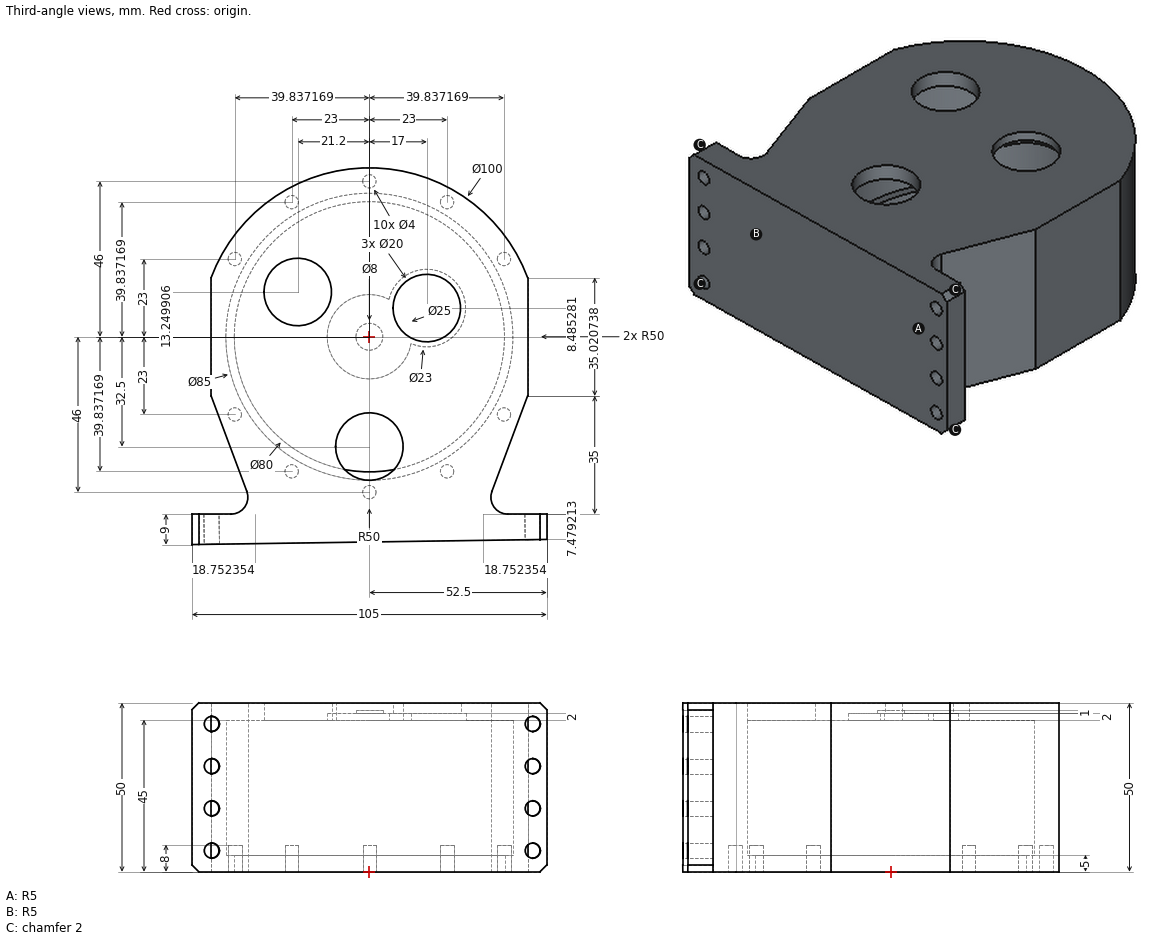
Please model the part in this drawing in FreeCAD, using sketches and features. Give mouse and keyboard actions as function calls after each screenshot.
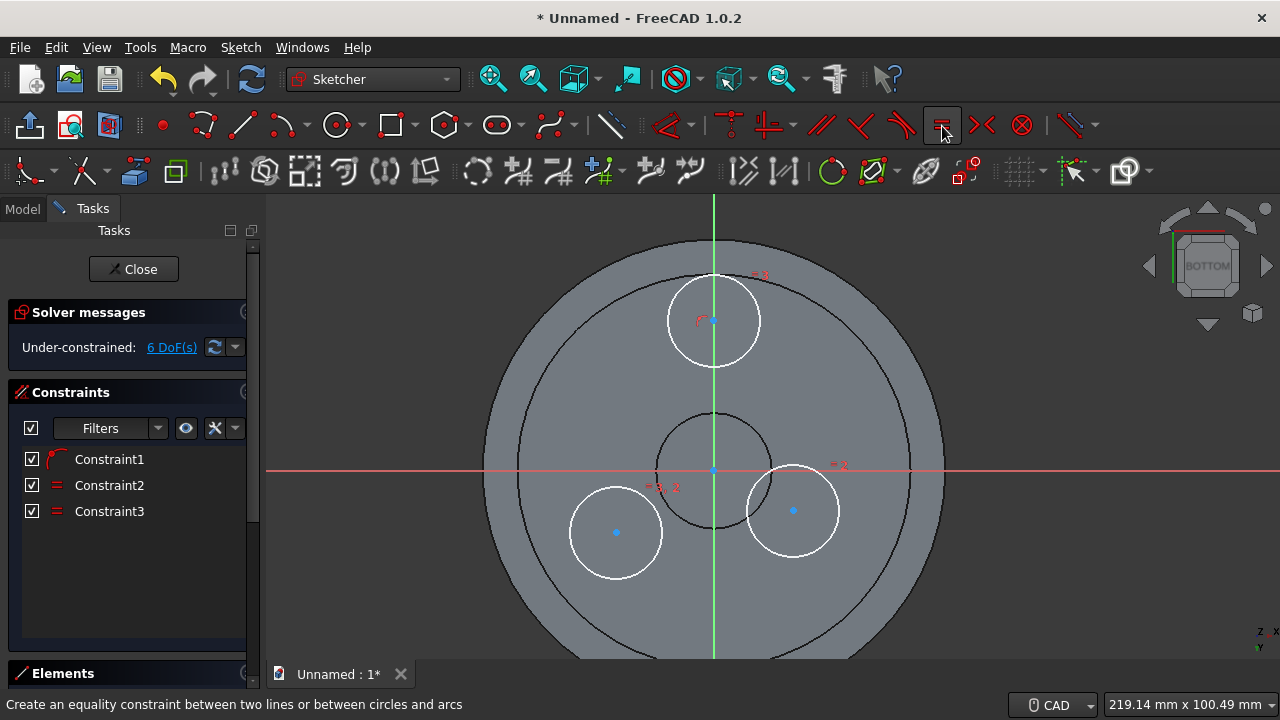
click(666, 126)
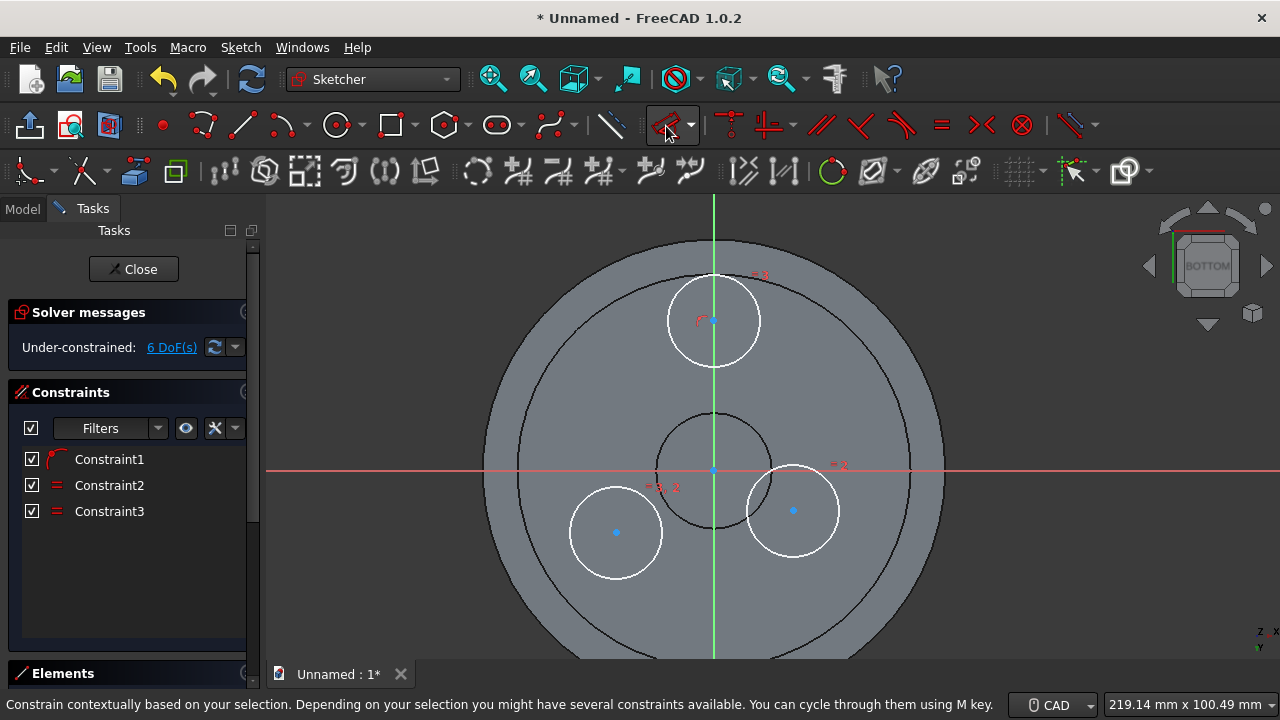
click(761, 544)
click(739, 567)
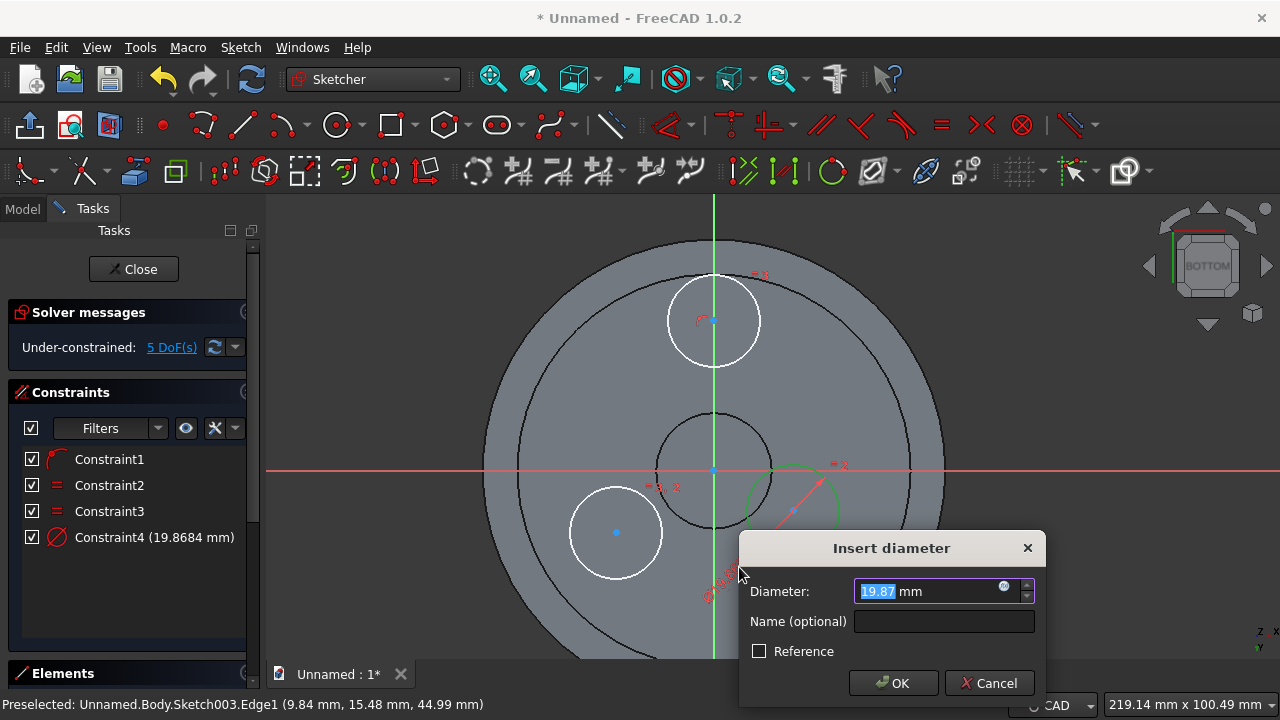
text(20)
key(Return)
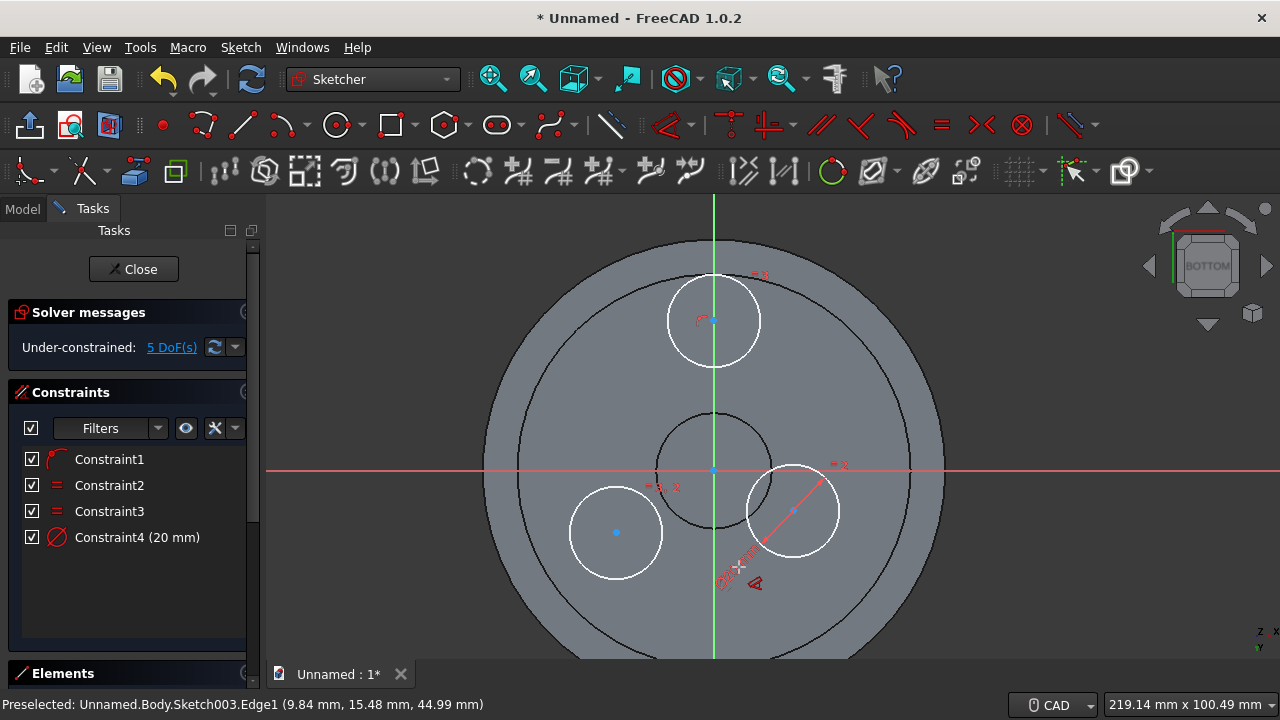
click(793, 511)
click(735, 545)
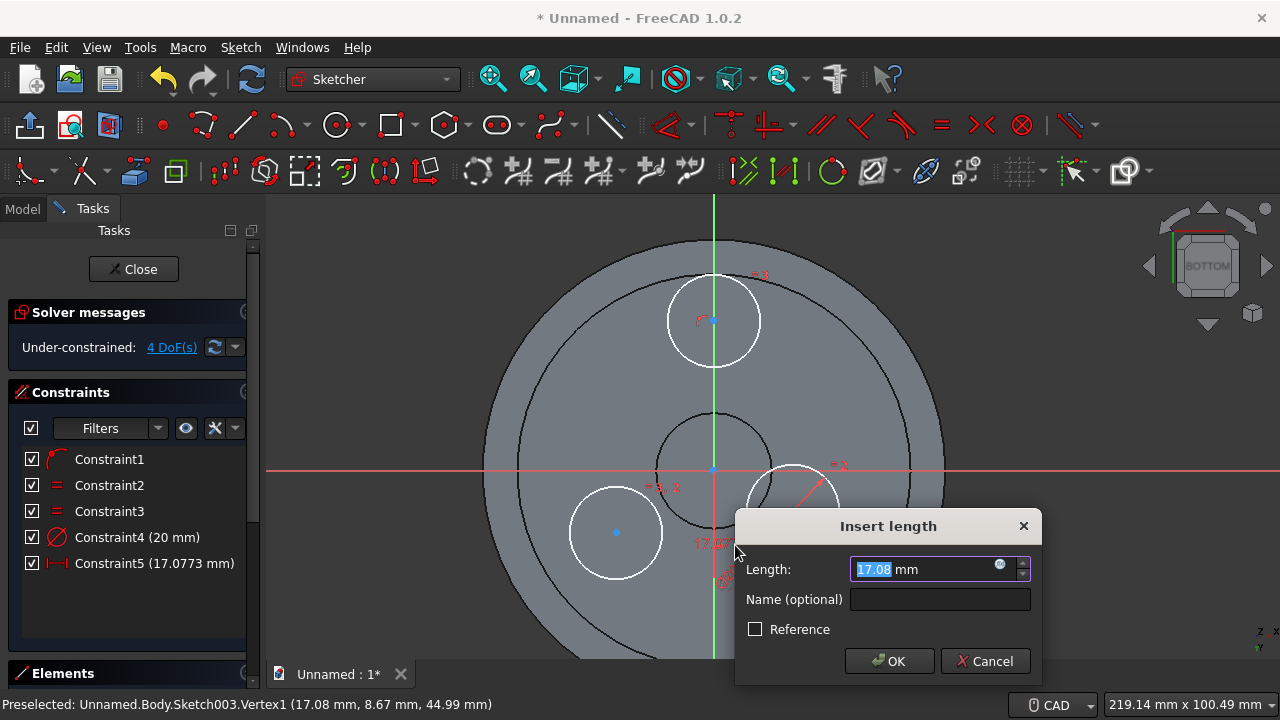
text(17)
key(Return)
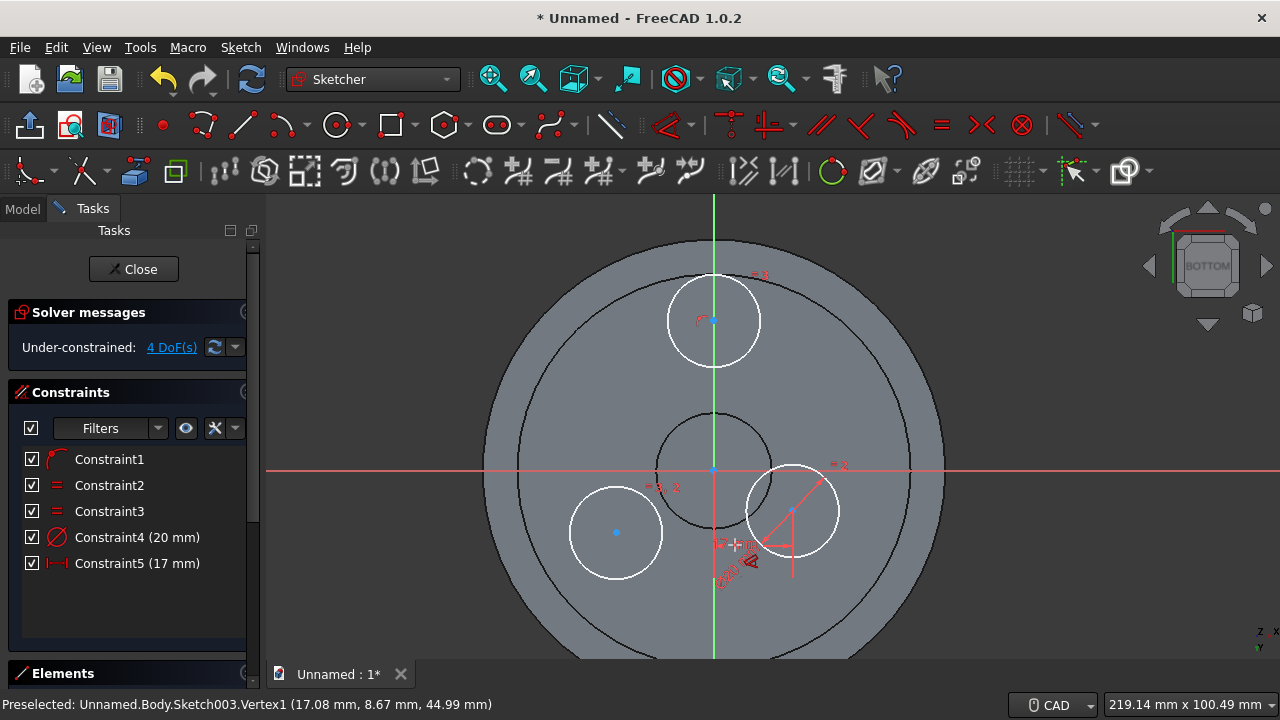
click(616, 533)
click(665, 567)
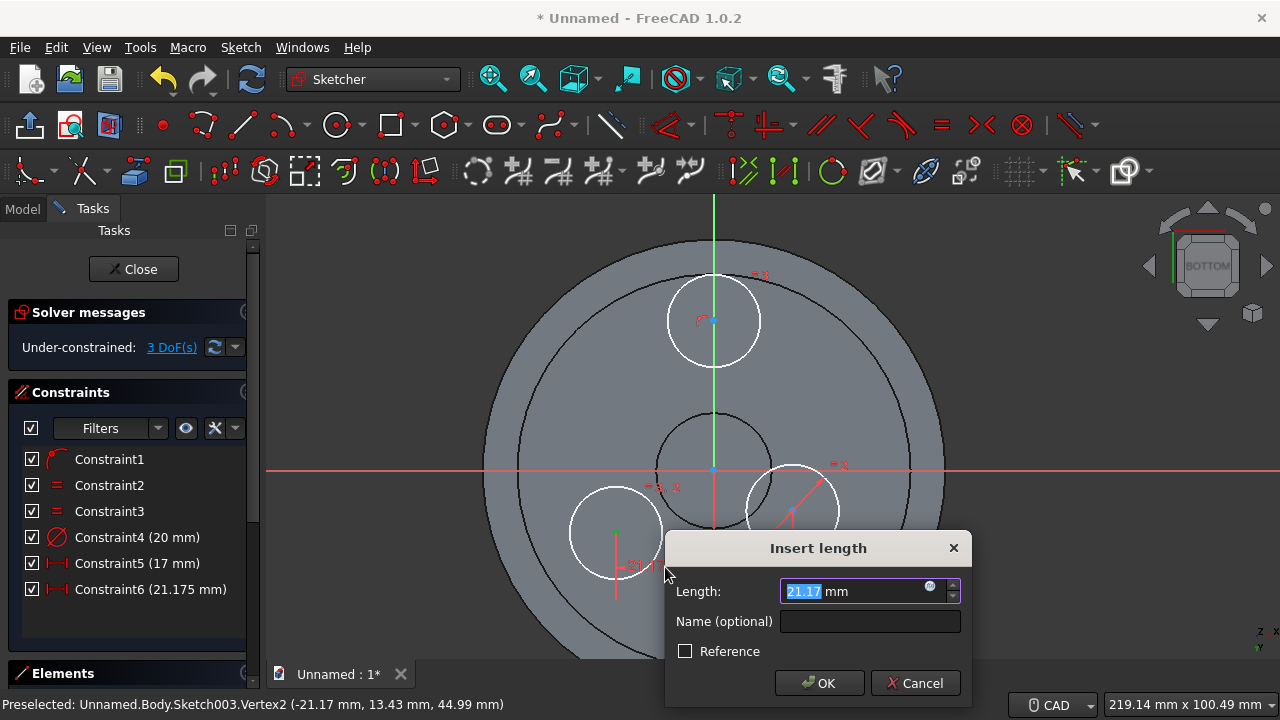
text(21.2)
key(Return)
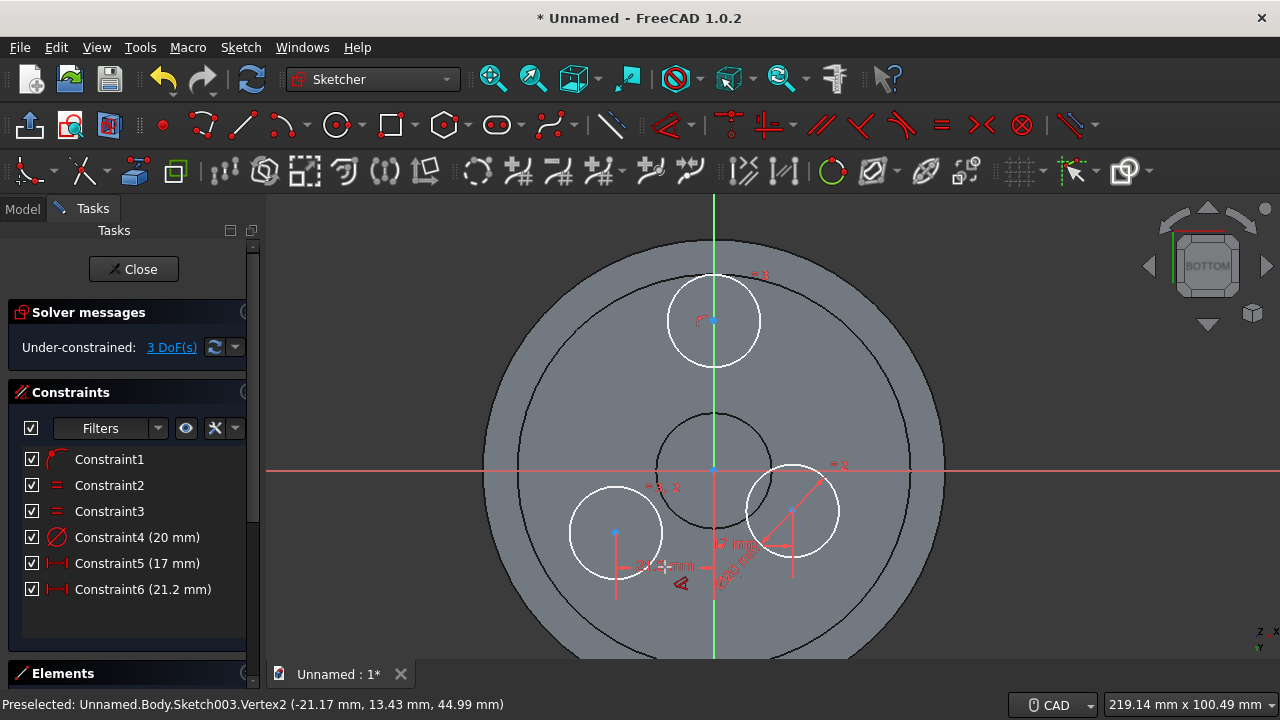
click(714, 321)
click(748, 396)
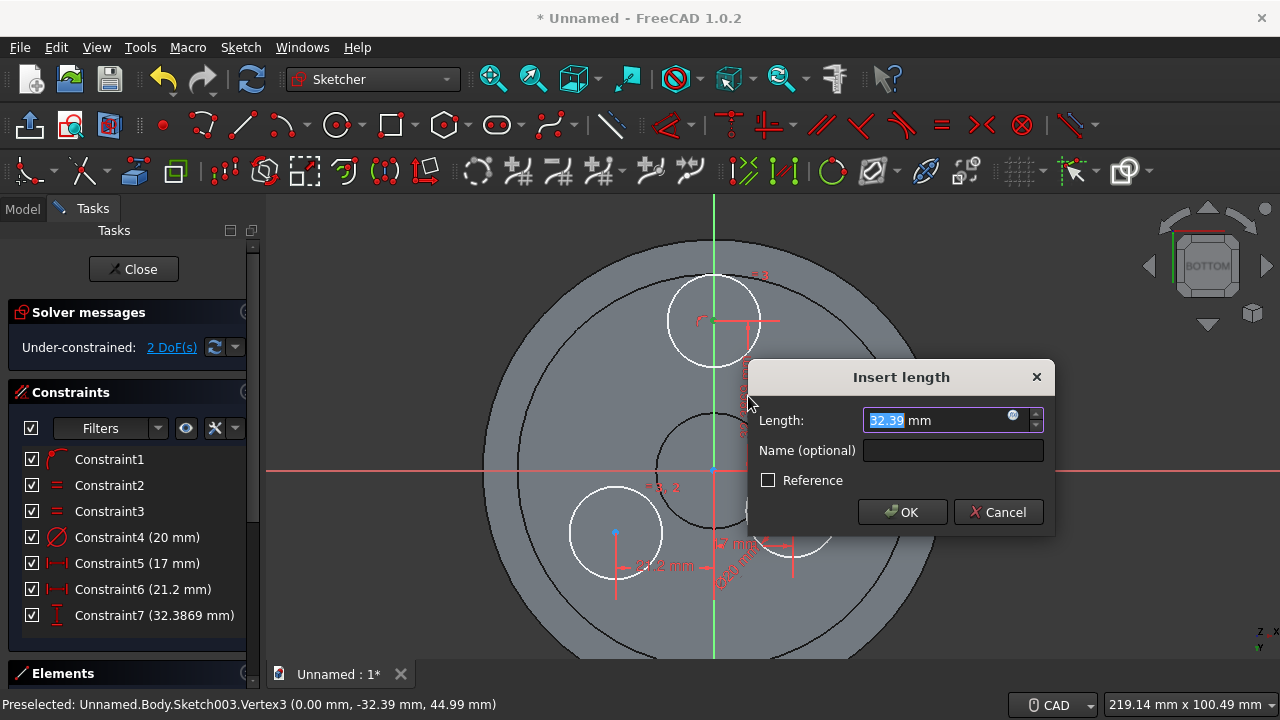
text(32.5)
key(Return)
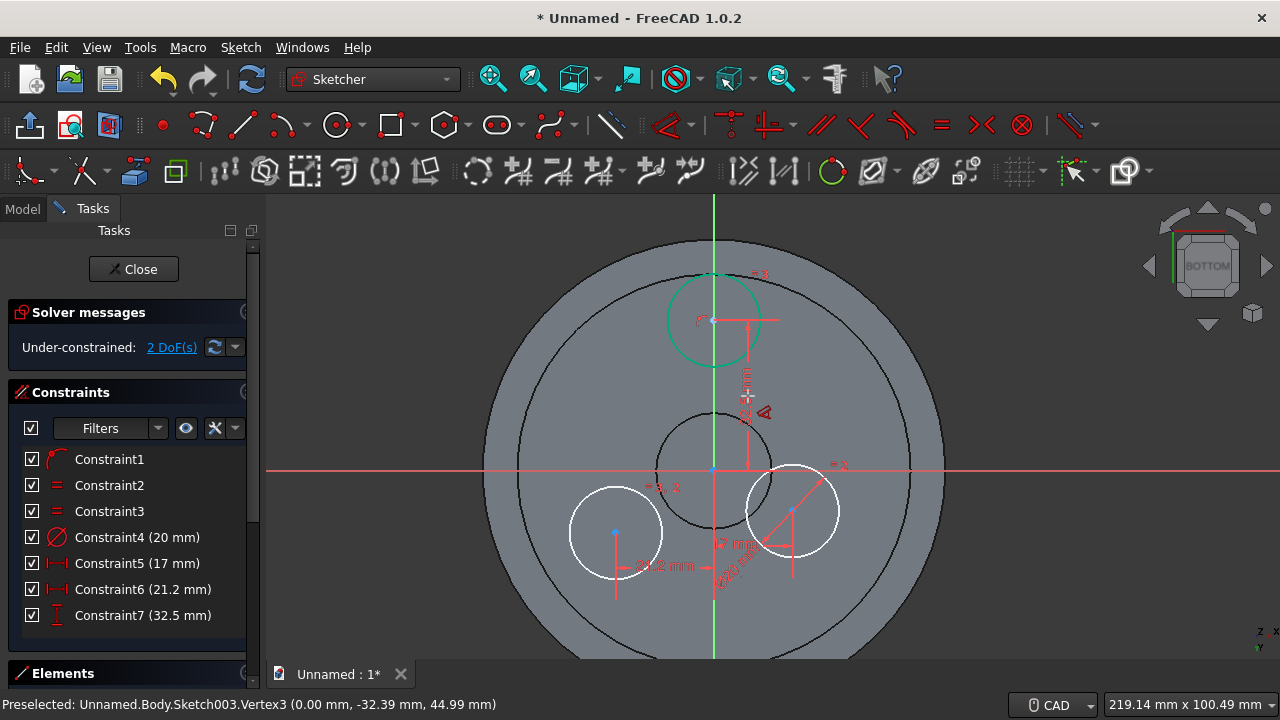
click(793, 511)
click(680, 491)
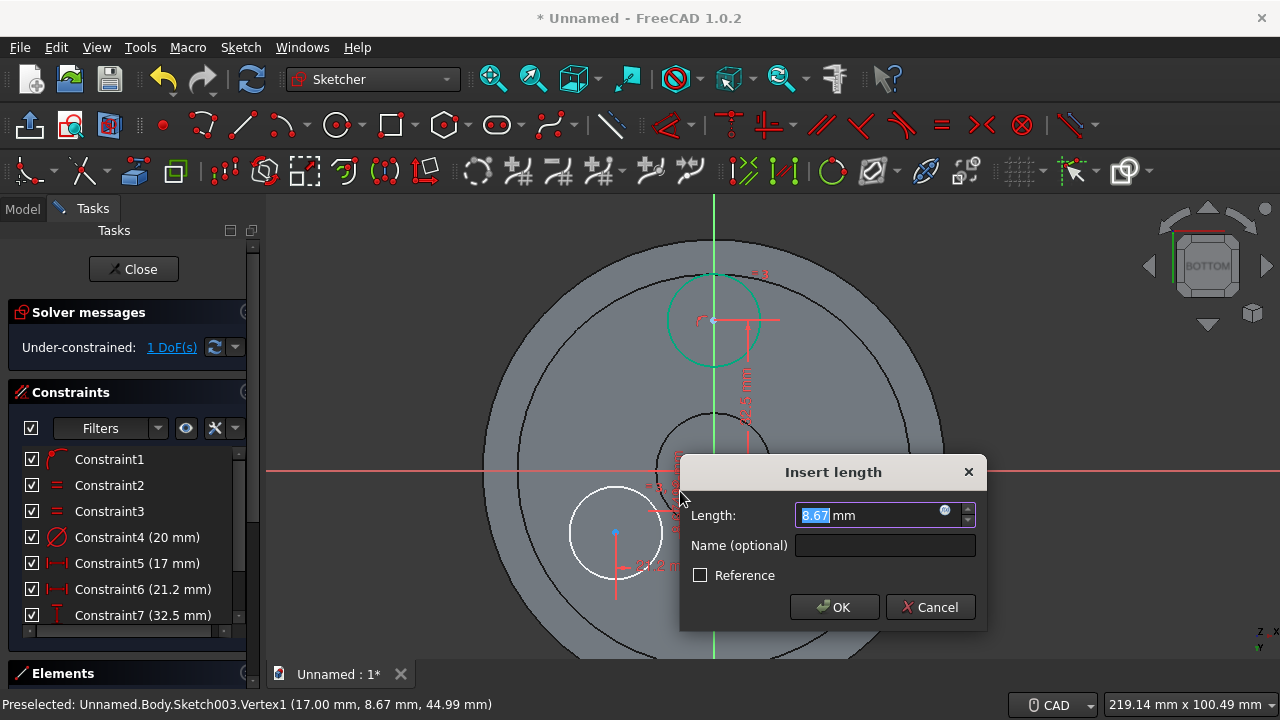
text(8.485281)
key(Return)